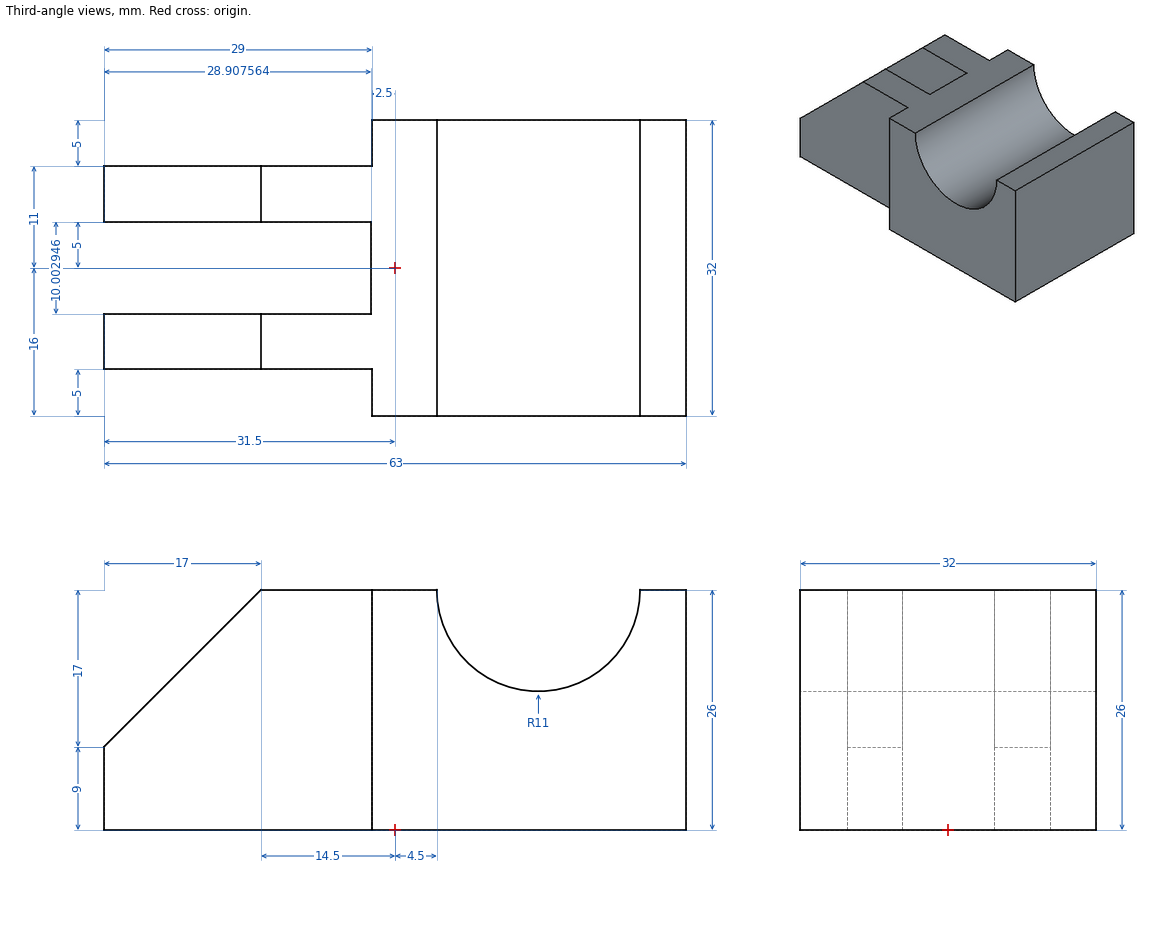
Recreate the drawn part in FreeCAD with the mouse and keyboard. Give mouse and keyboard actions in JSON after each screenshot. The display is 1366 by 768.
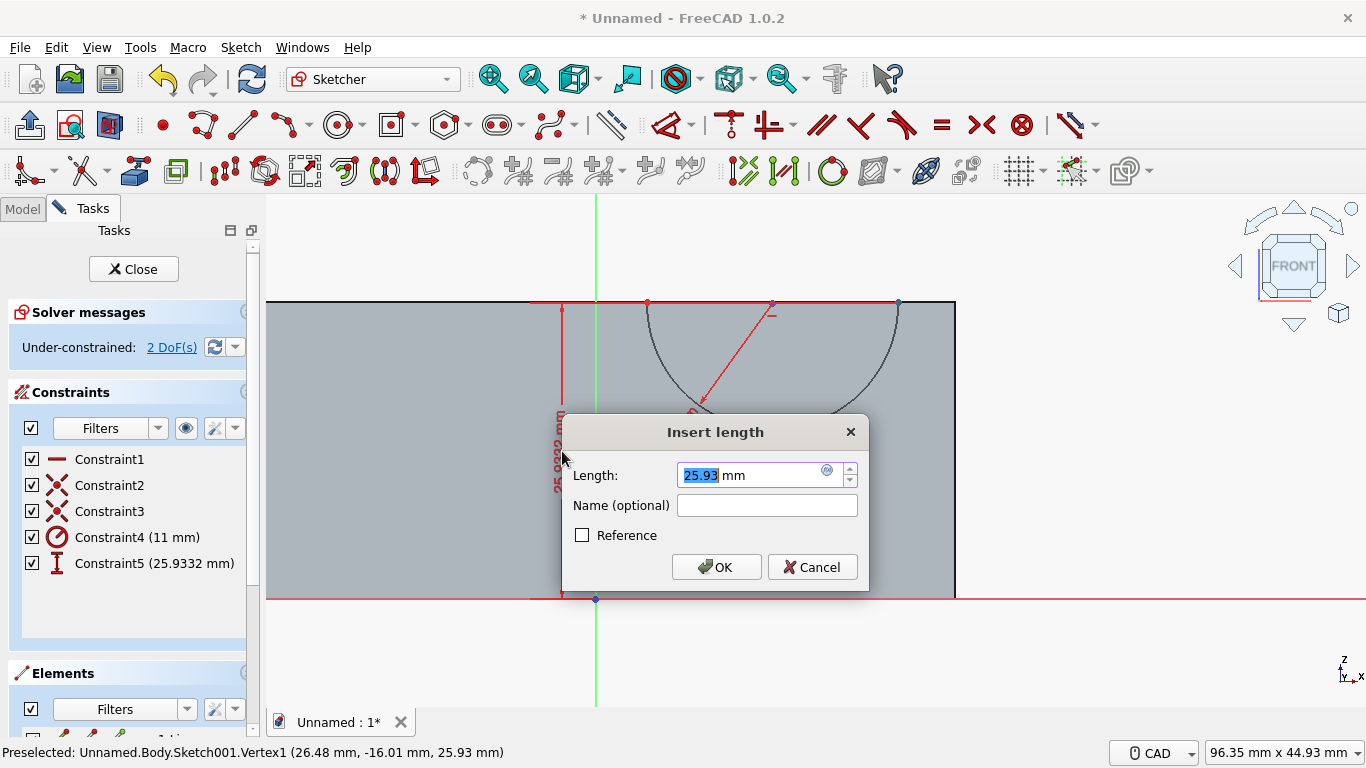
{"action": "type", "text": "26"}
{"action": "key", "text": "Return"}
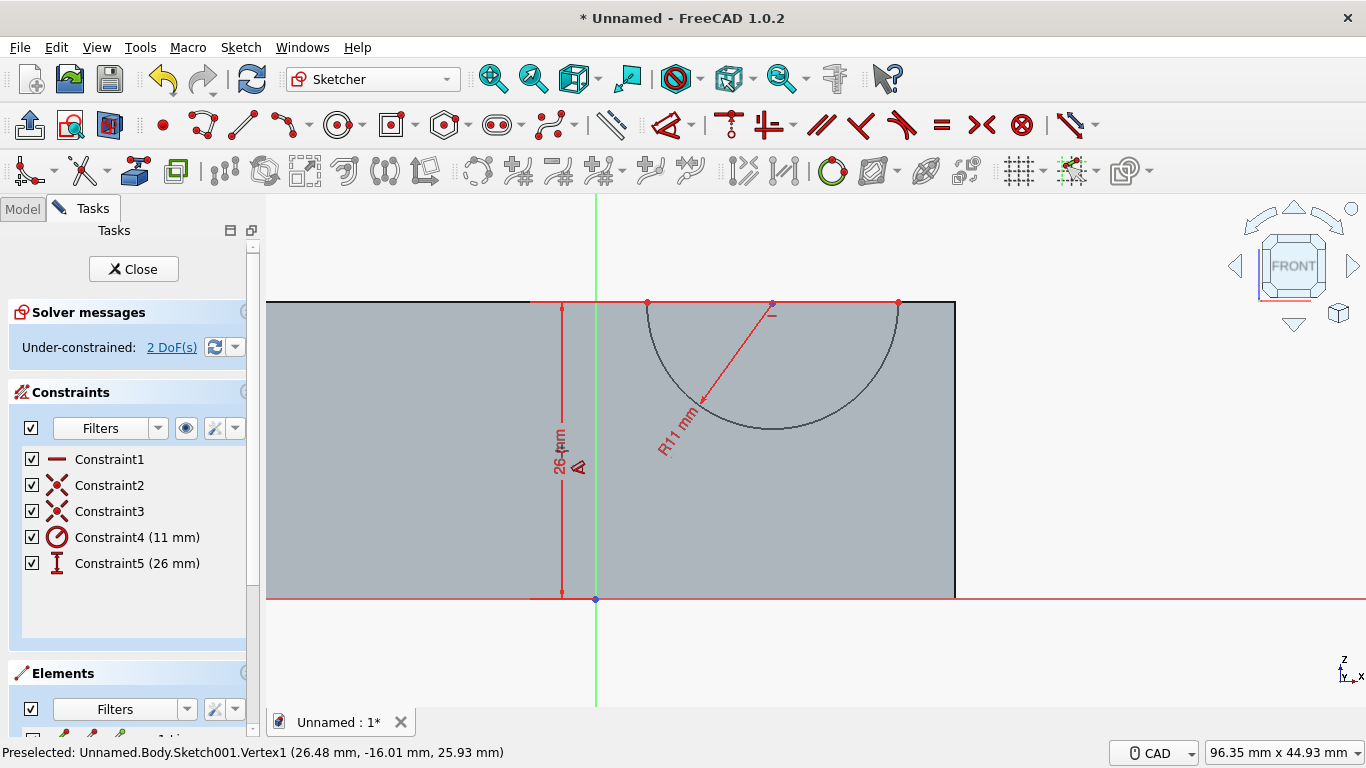
{"action": "left_click", "coordinate": [773, 303]}
{"action": "left_click", "coordinate": [562, 383]}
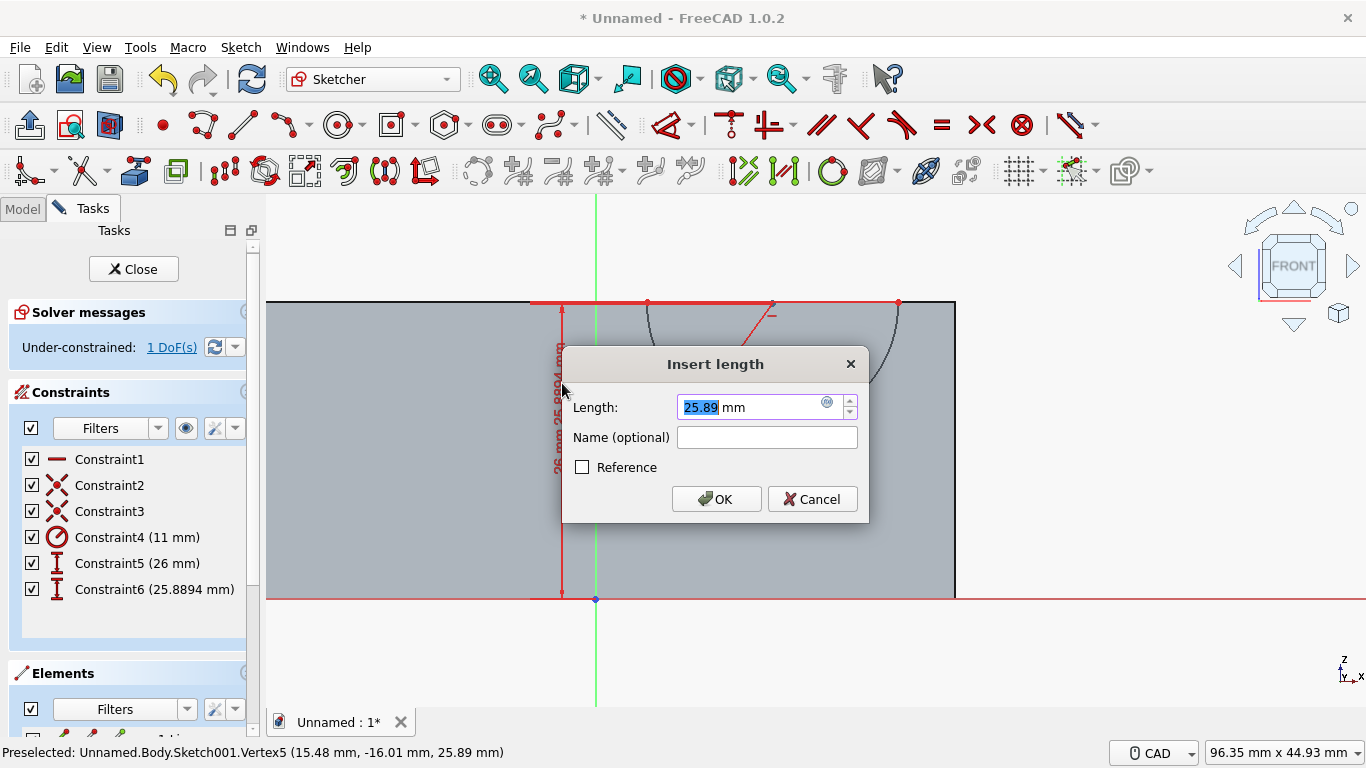
{"action": "type", "text": "26"}
{"action": "key", "text": "Return"}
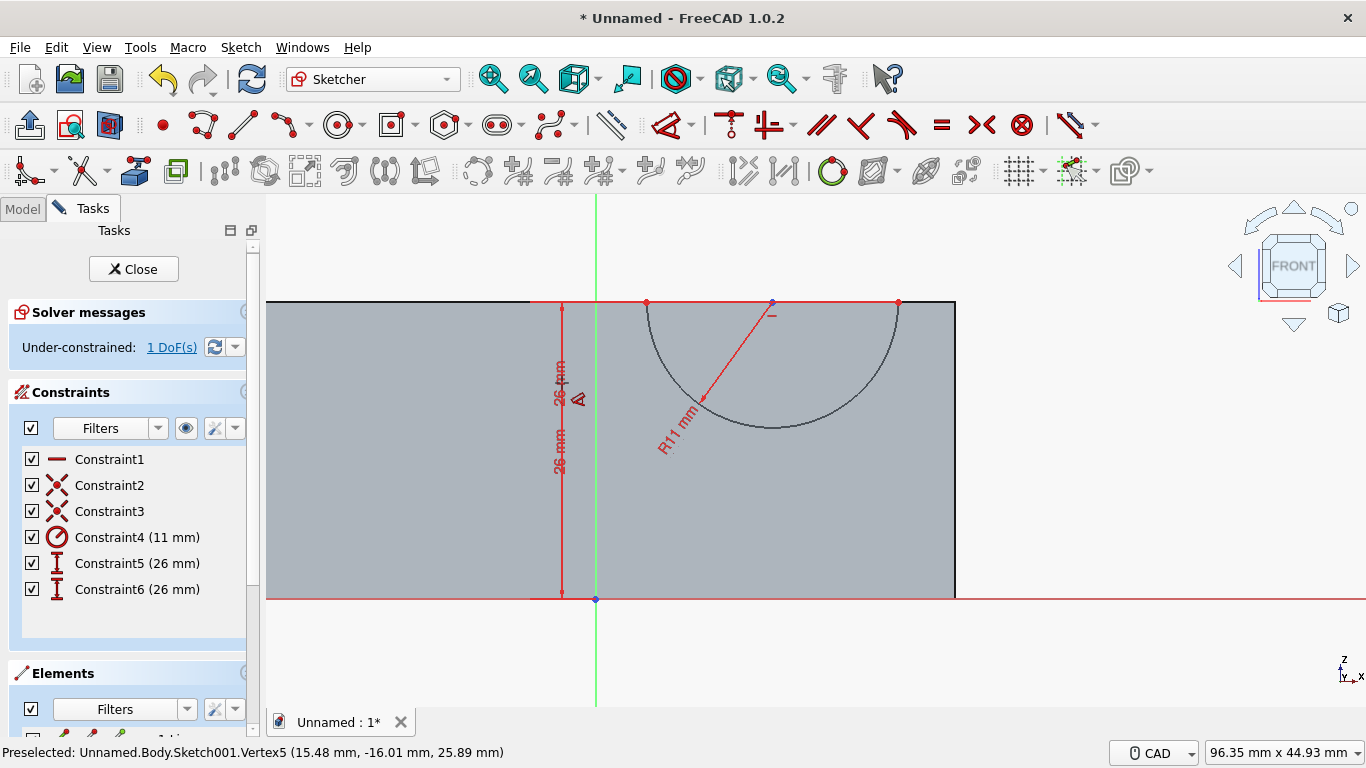
{"action": "left_click", "coordinate": [647, 302]}
{"action": "left_click", "coordinate": [621, 633]}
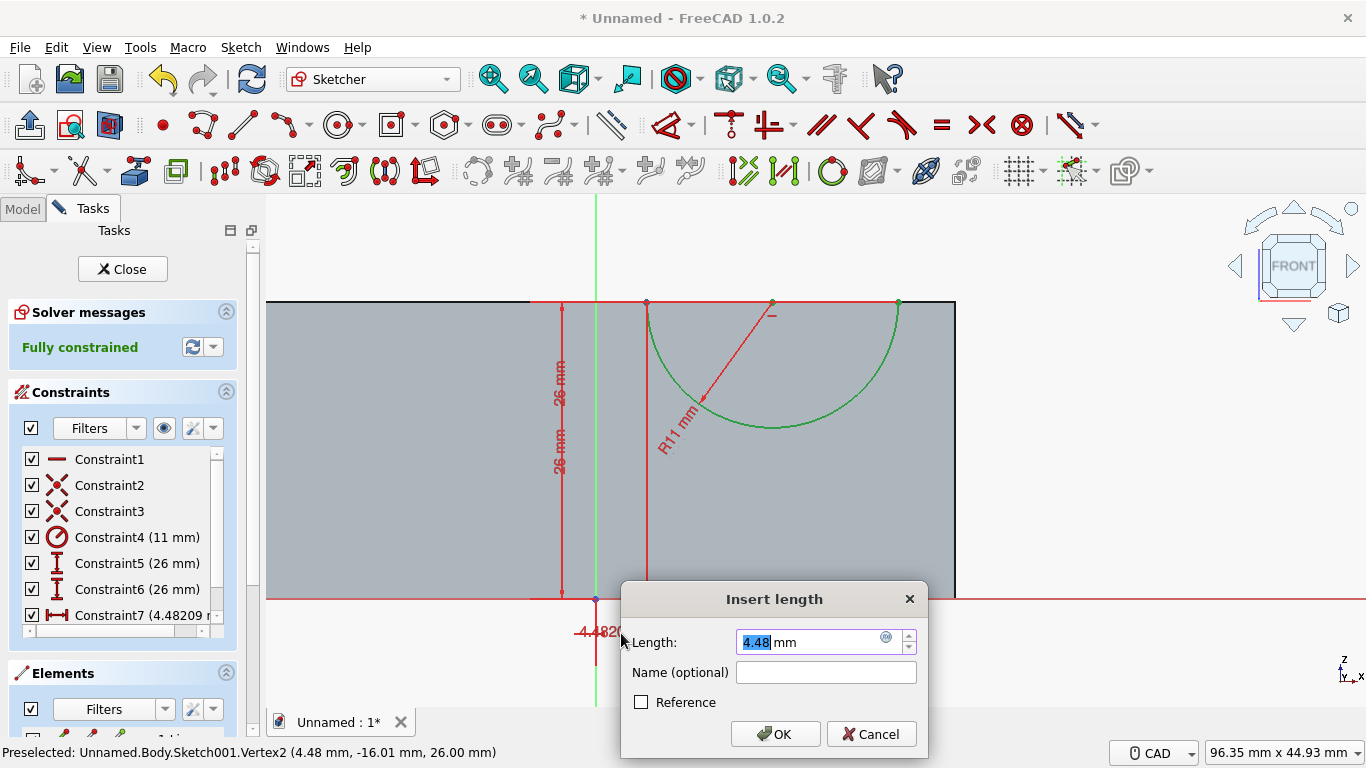
{"action": "type", "text": "4.5"}
{"action": "key", "text": "Return"}
{"action": "key", "text": "Escape"}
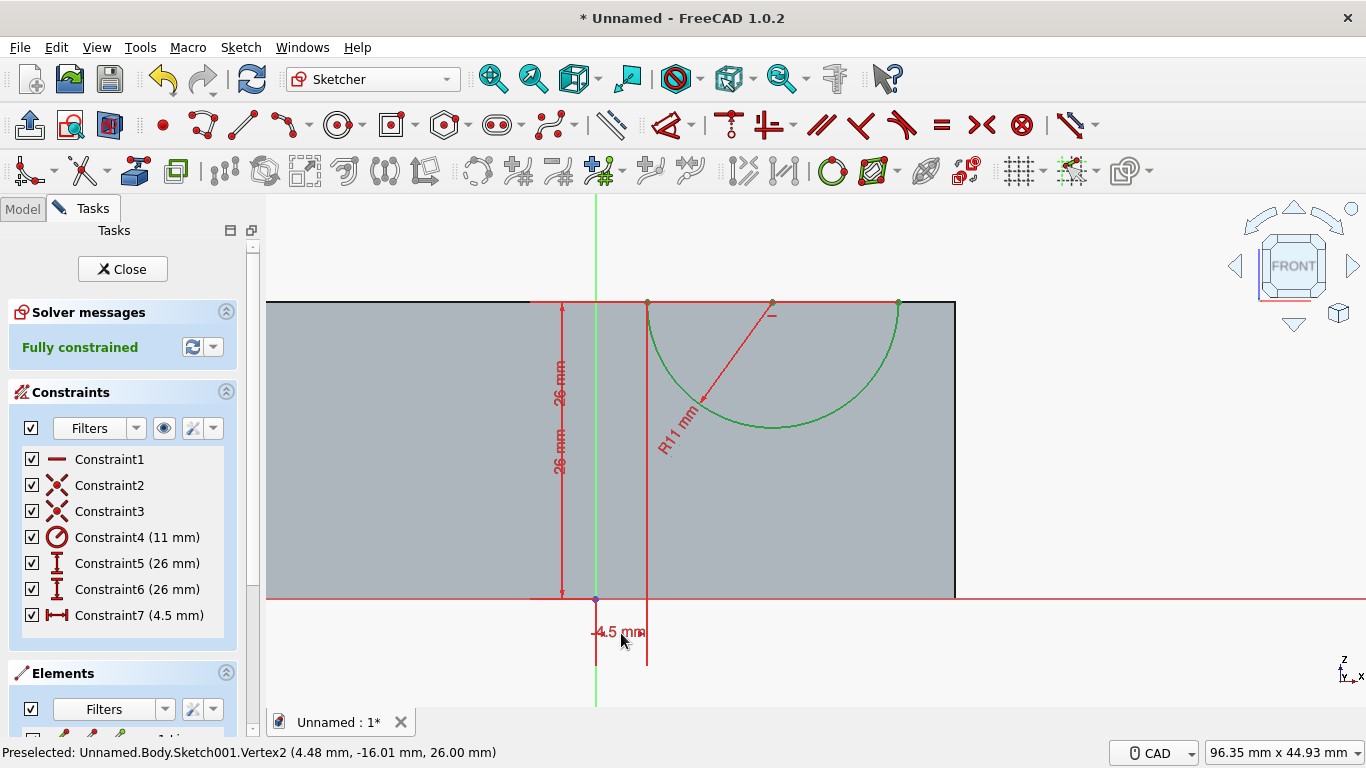
{"action": "left_click", "coordinate": [123, 269]}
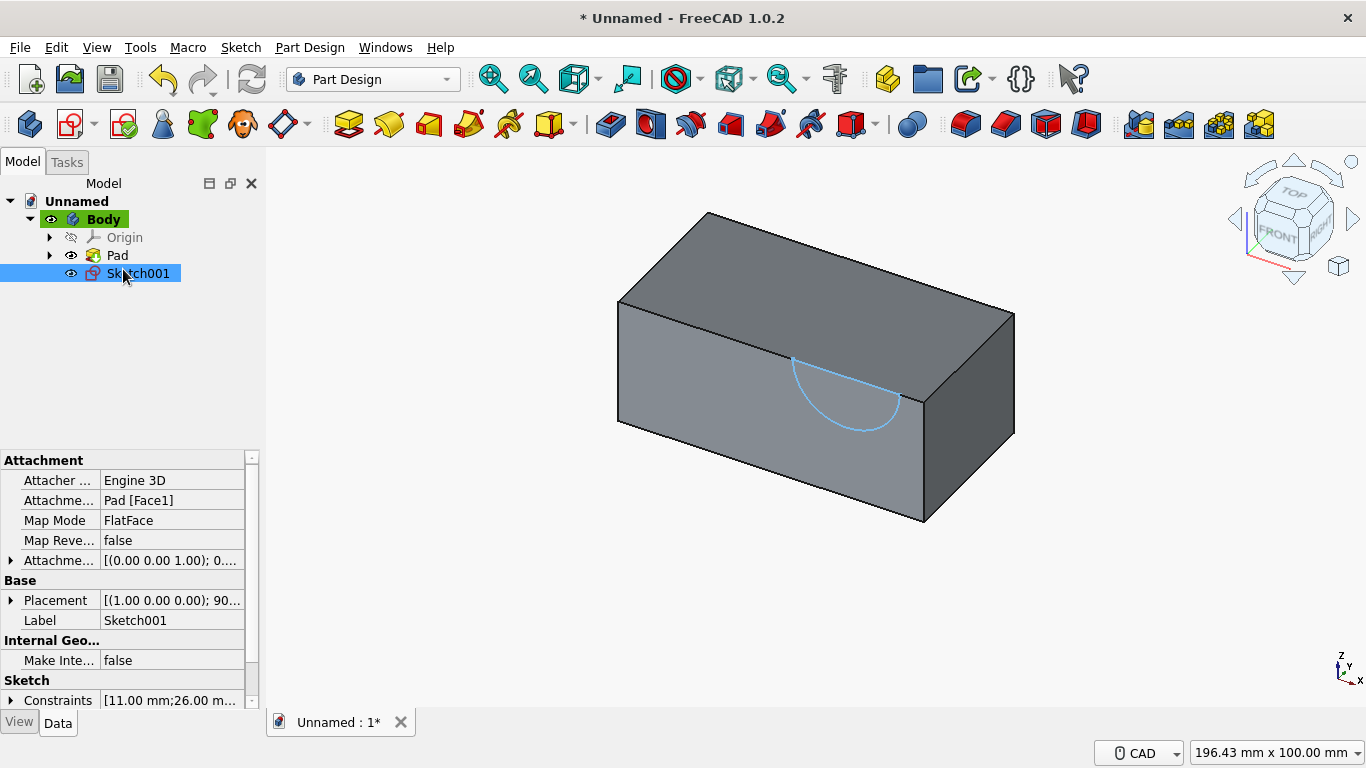
{"action": "left_click", "coordinate": [612, 124]}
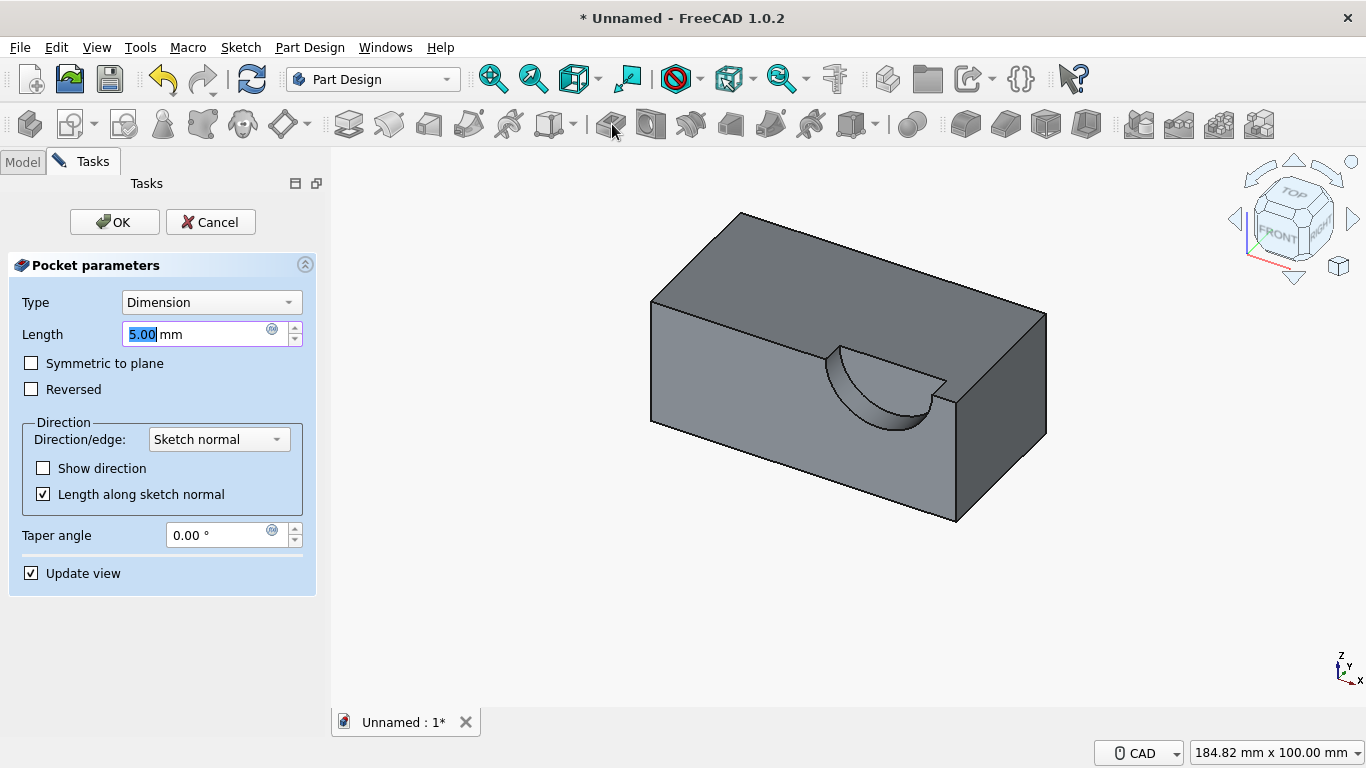
{"action": "type", "text": "32"}
{"action": "key", "text": "Tab"}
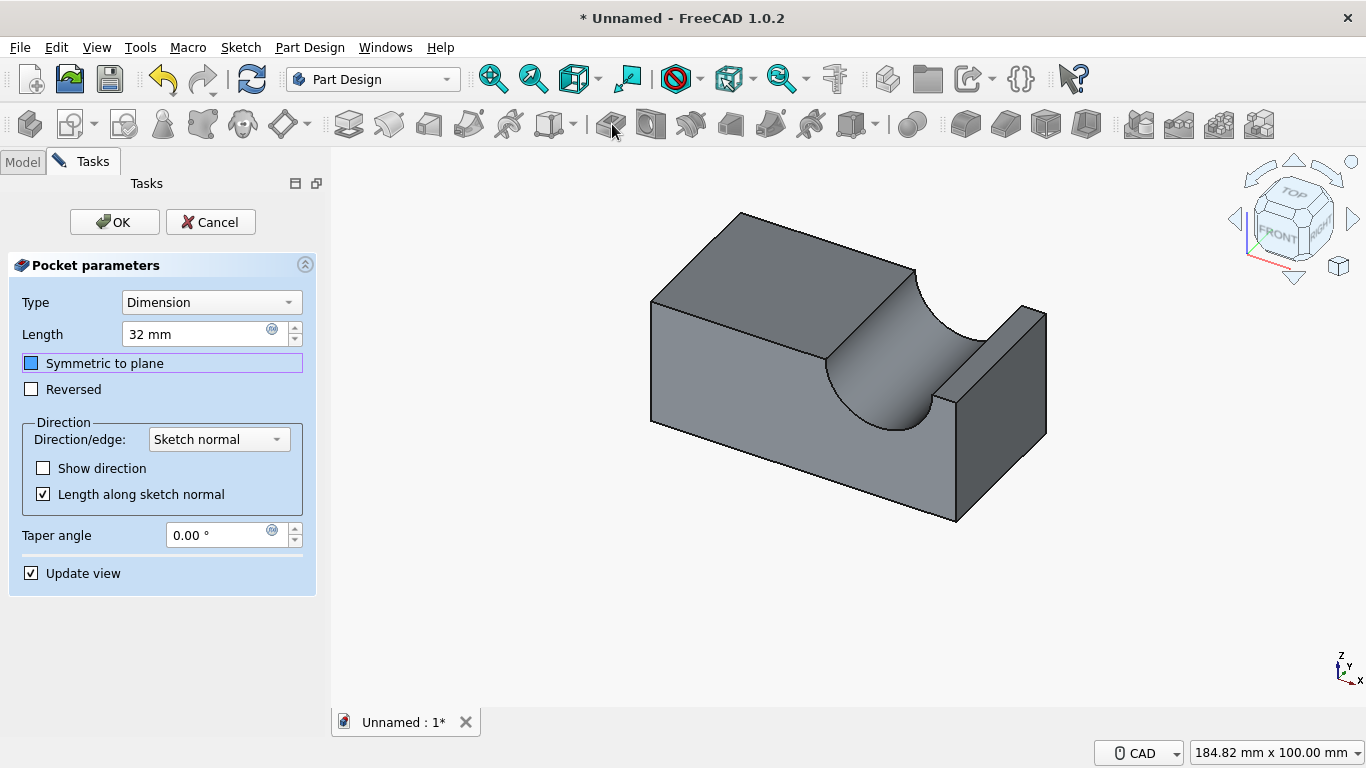
{"action": "left_click", "coordinate": [115, 222]}